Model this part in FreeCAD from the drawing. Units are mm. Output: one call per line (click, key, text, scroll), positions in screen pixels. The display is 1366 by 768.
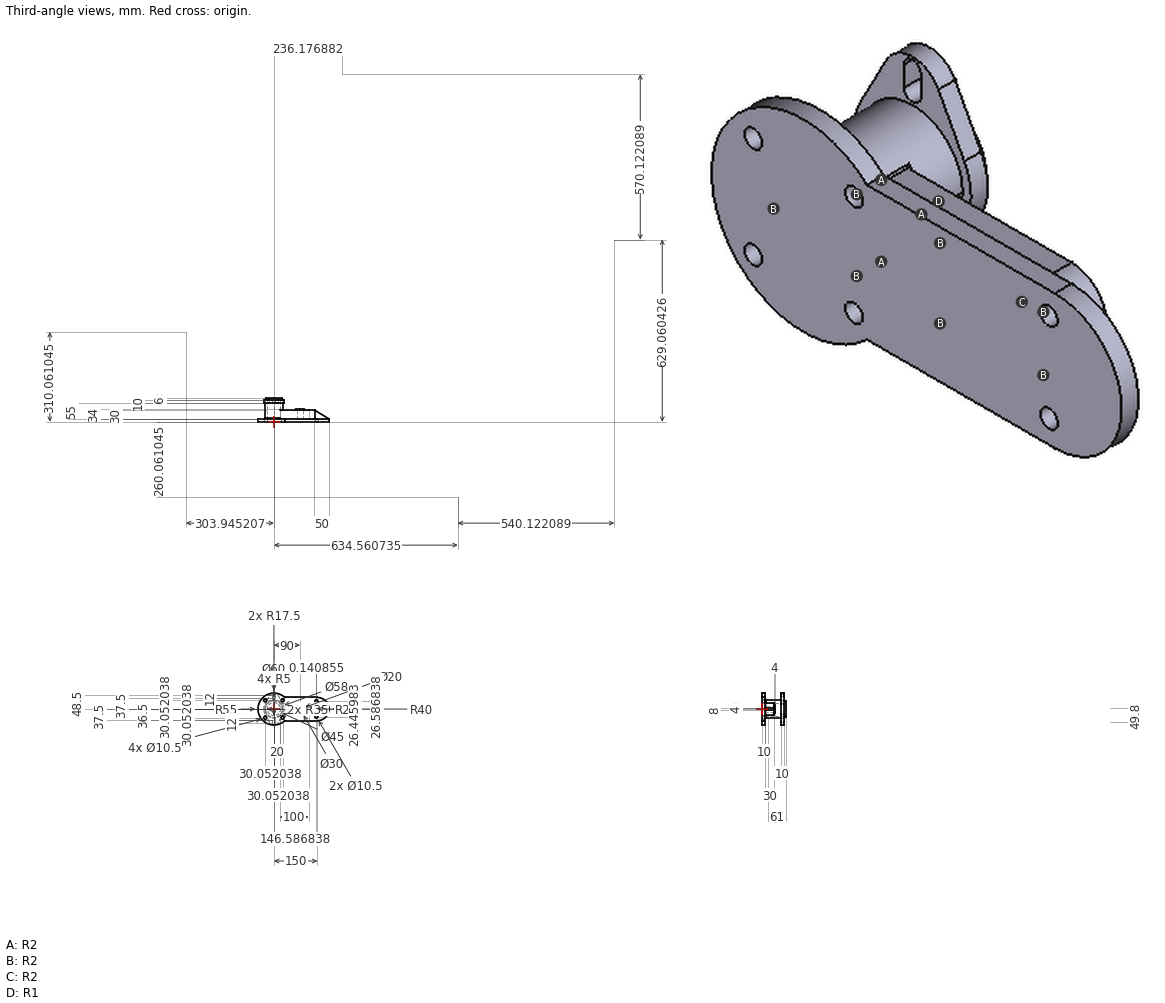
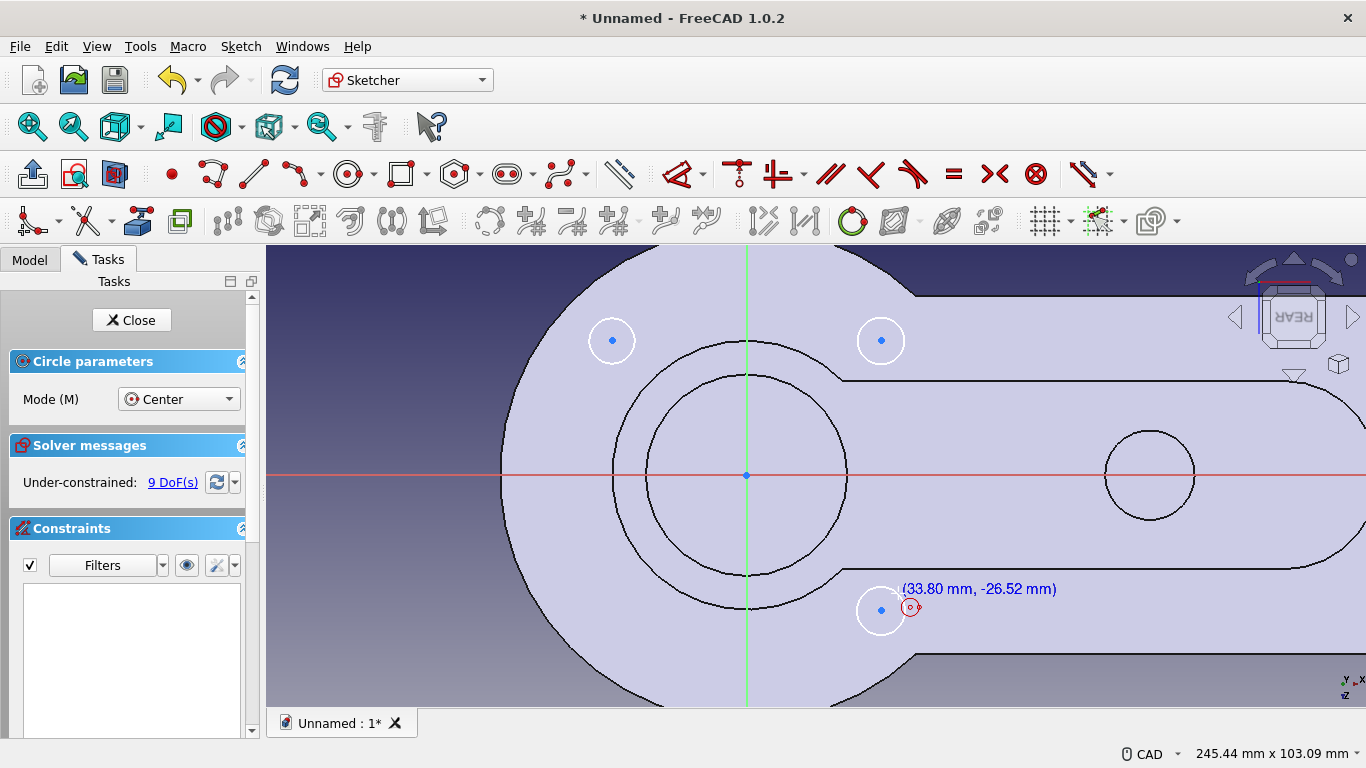
click(612, 610)
click(628, 593)
key(Escape)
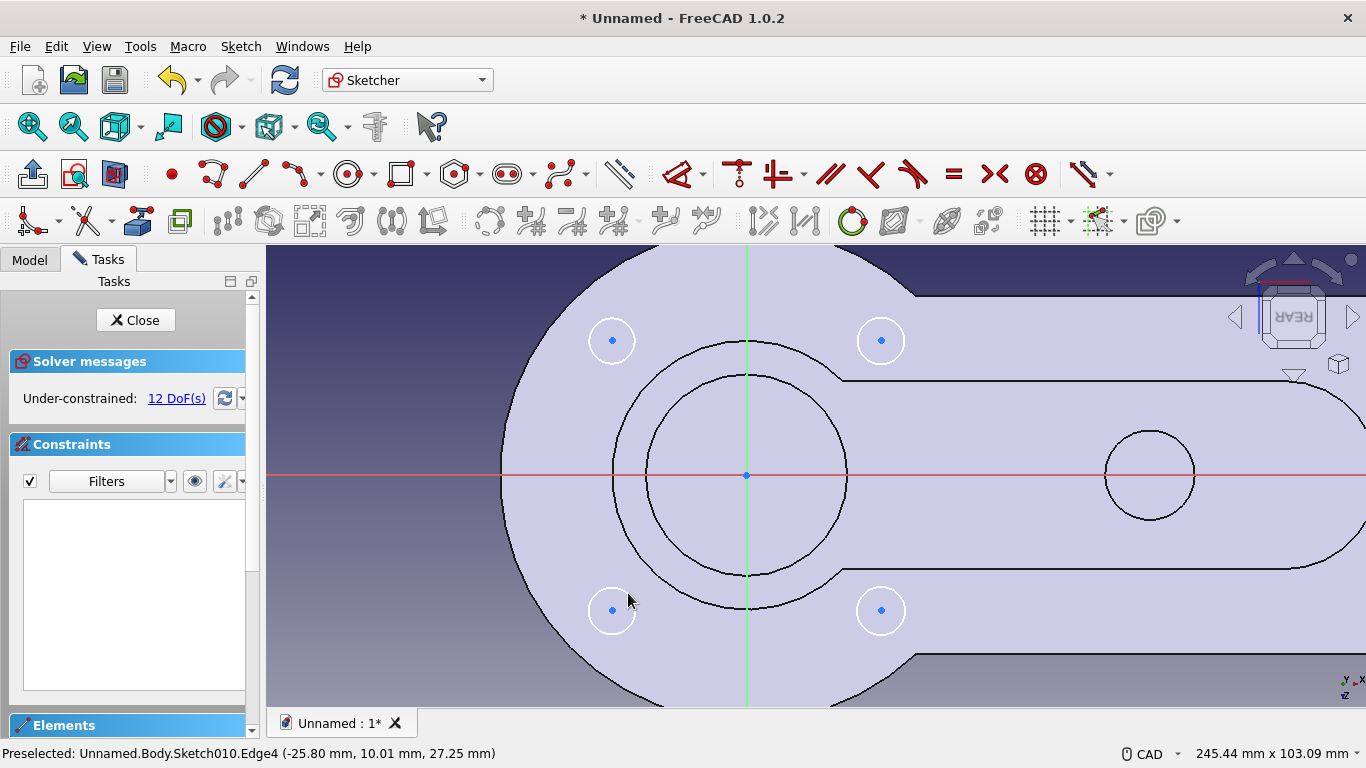
click(628, 325)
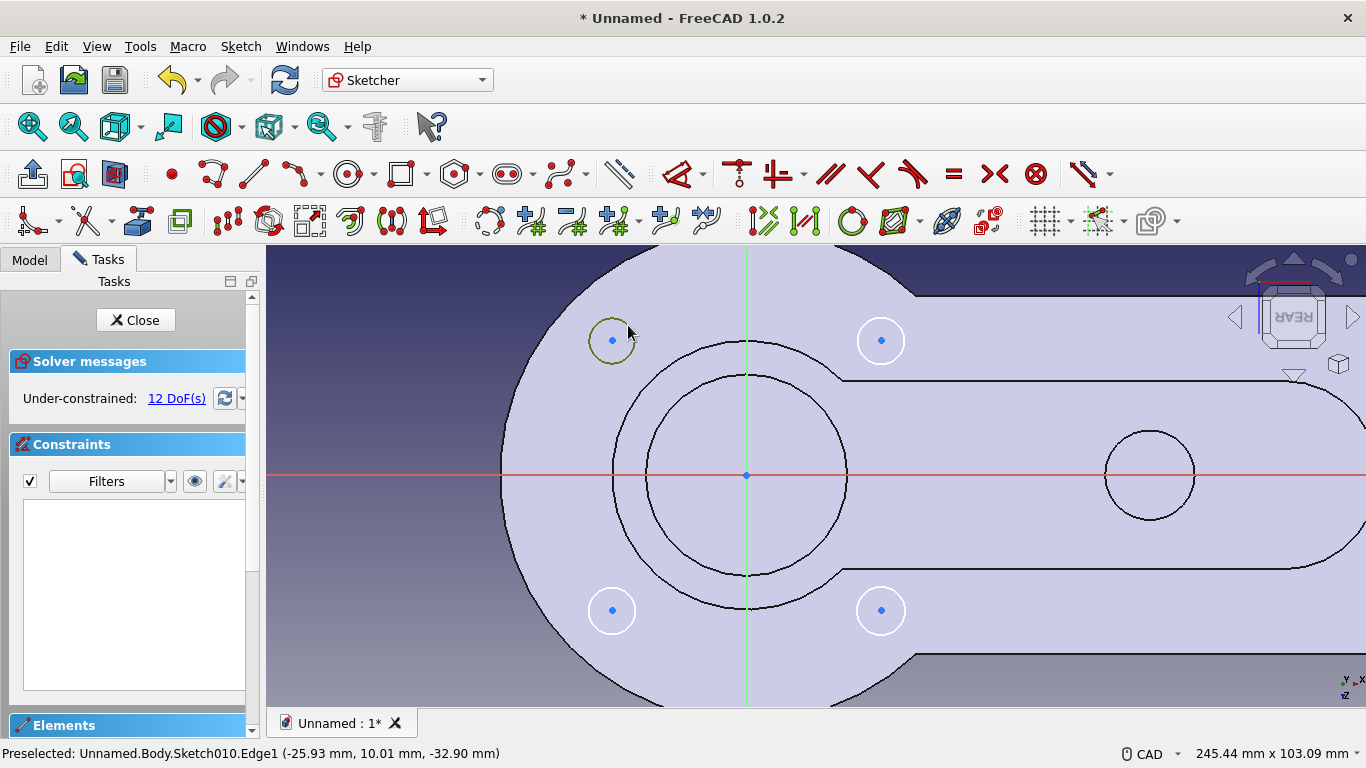
click(897, 324)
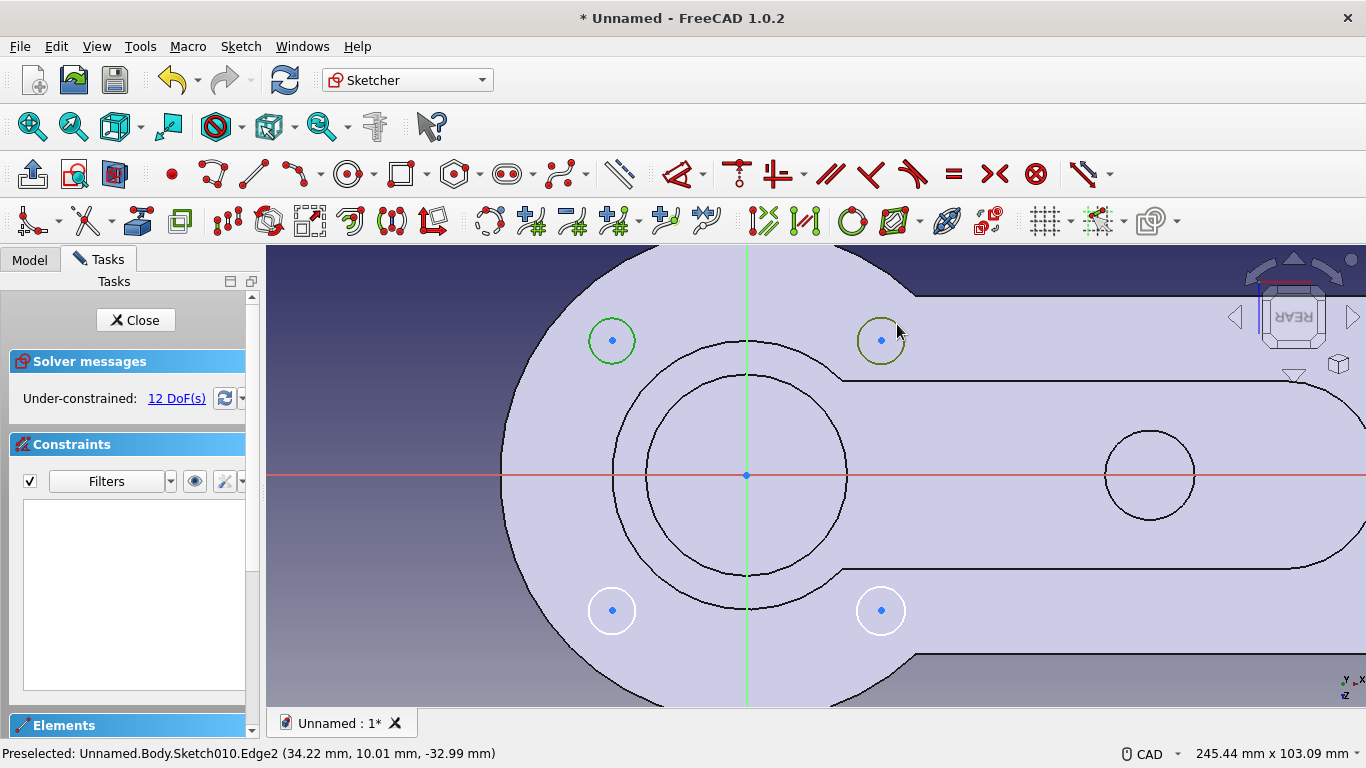
click(898, 594)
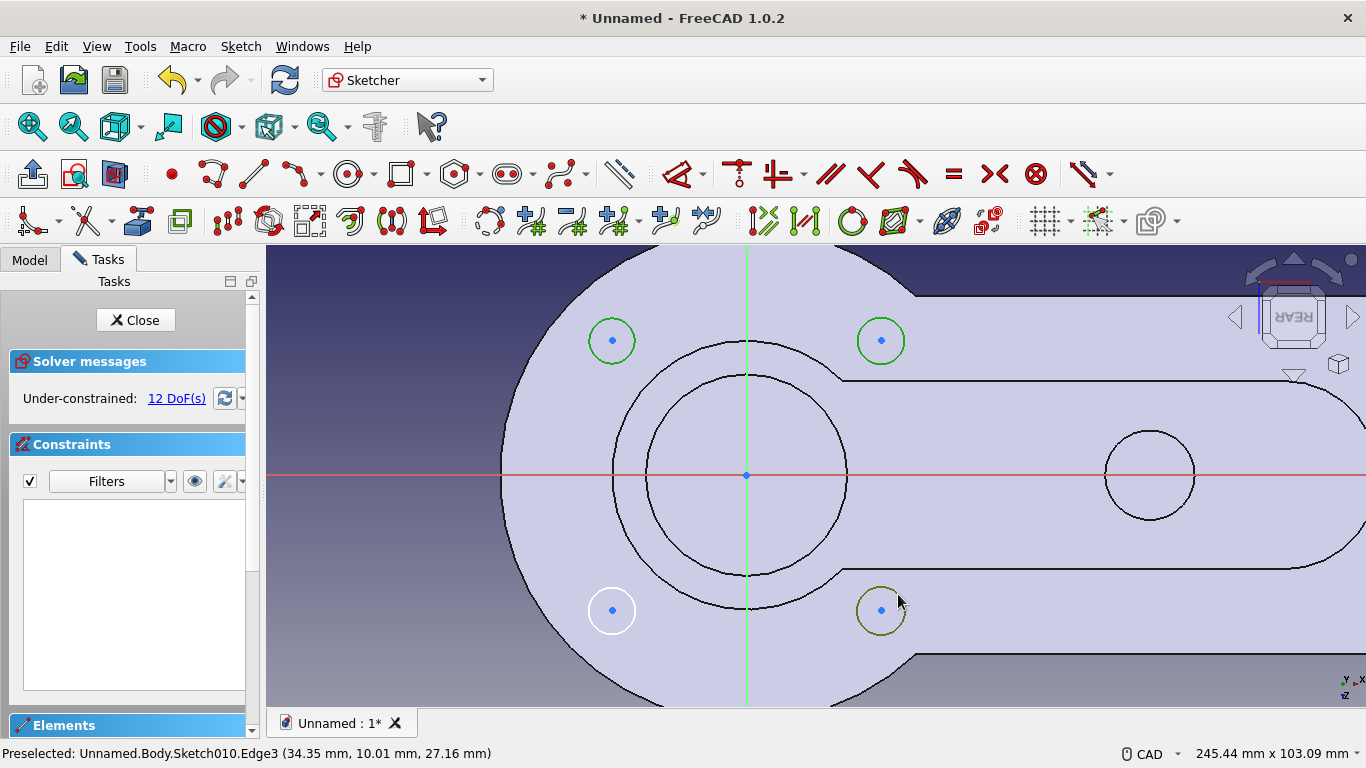
click(628, 594)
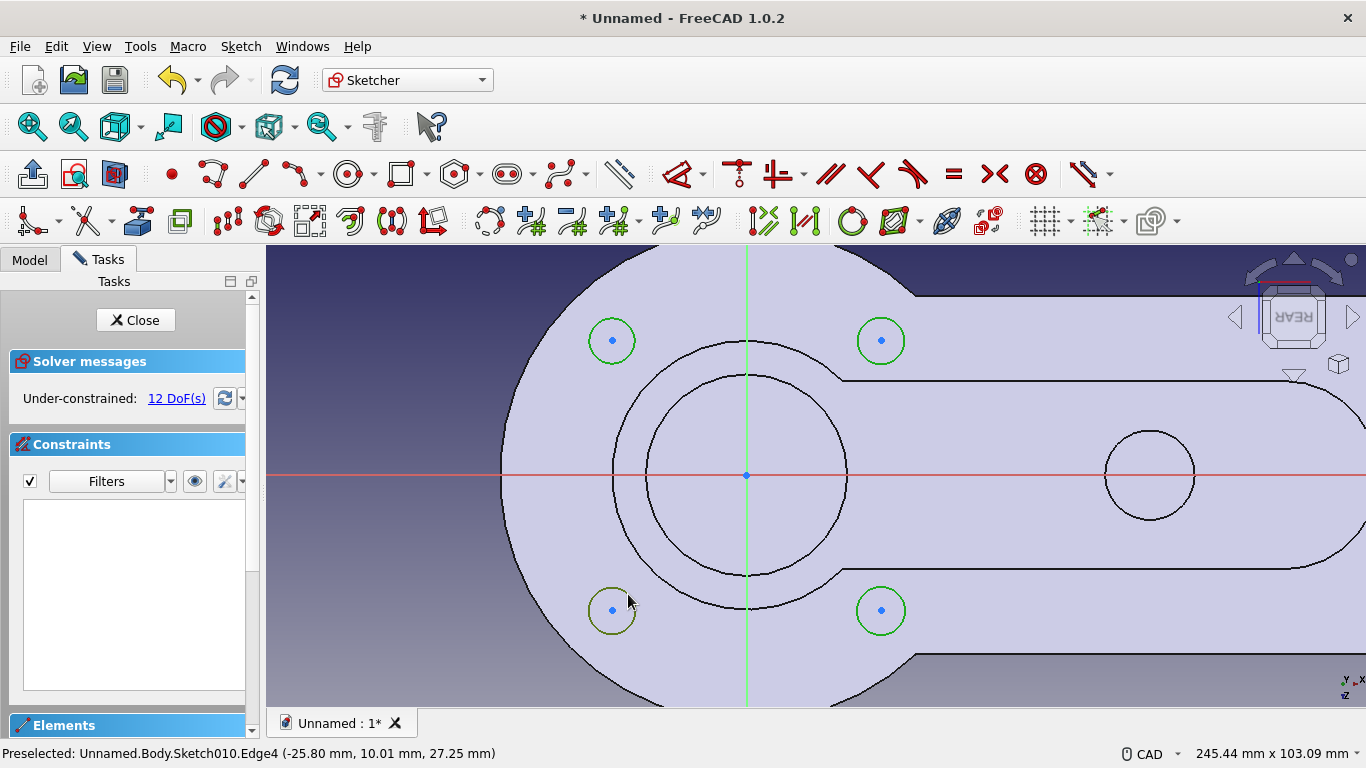
key(e)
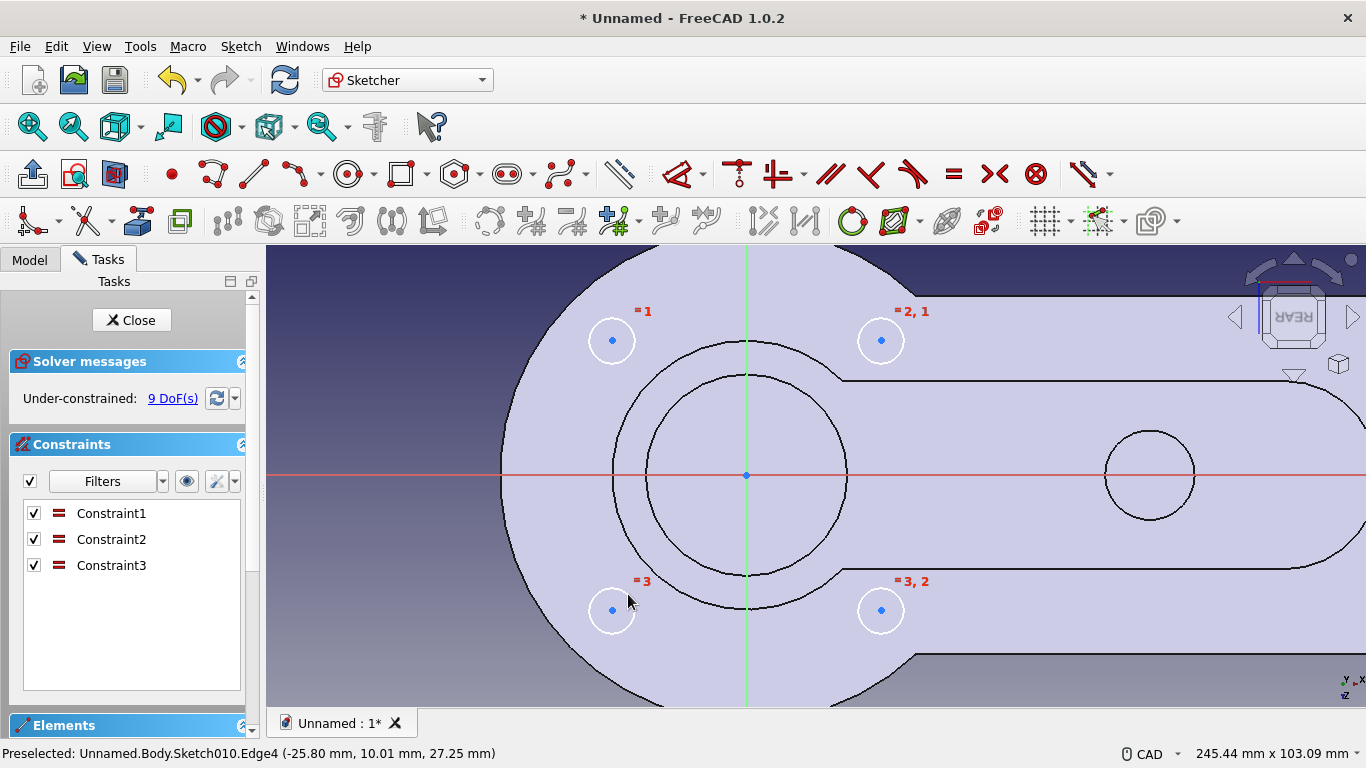
click(612, 341)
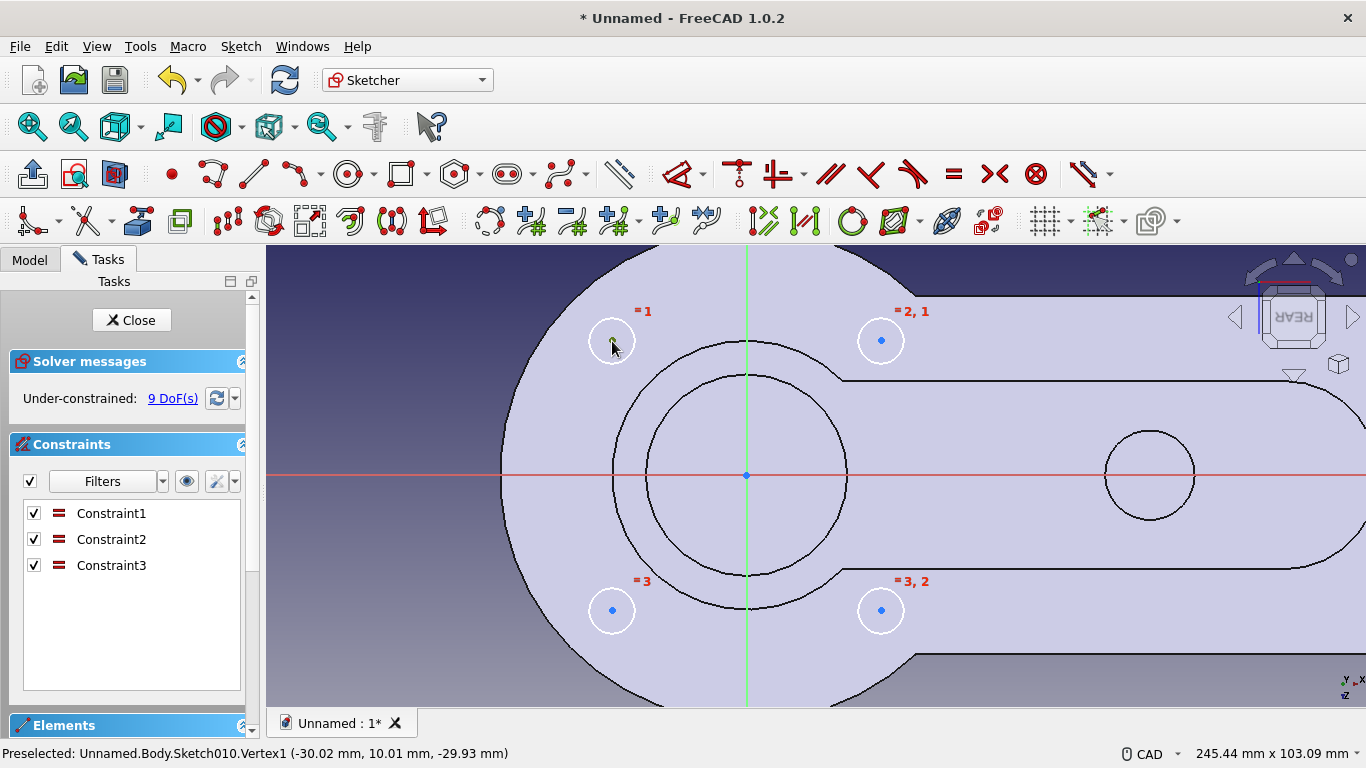
click(881, 341)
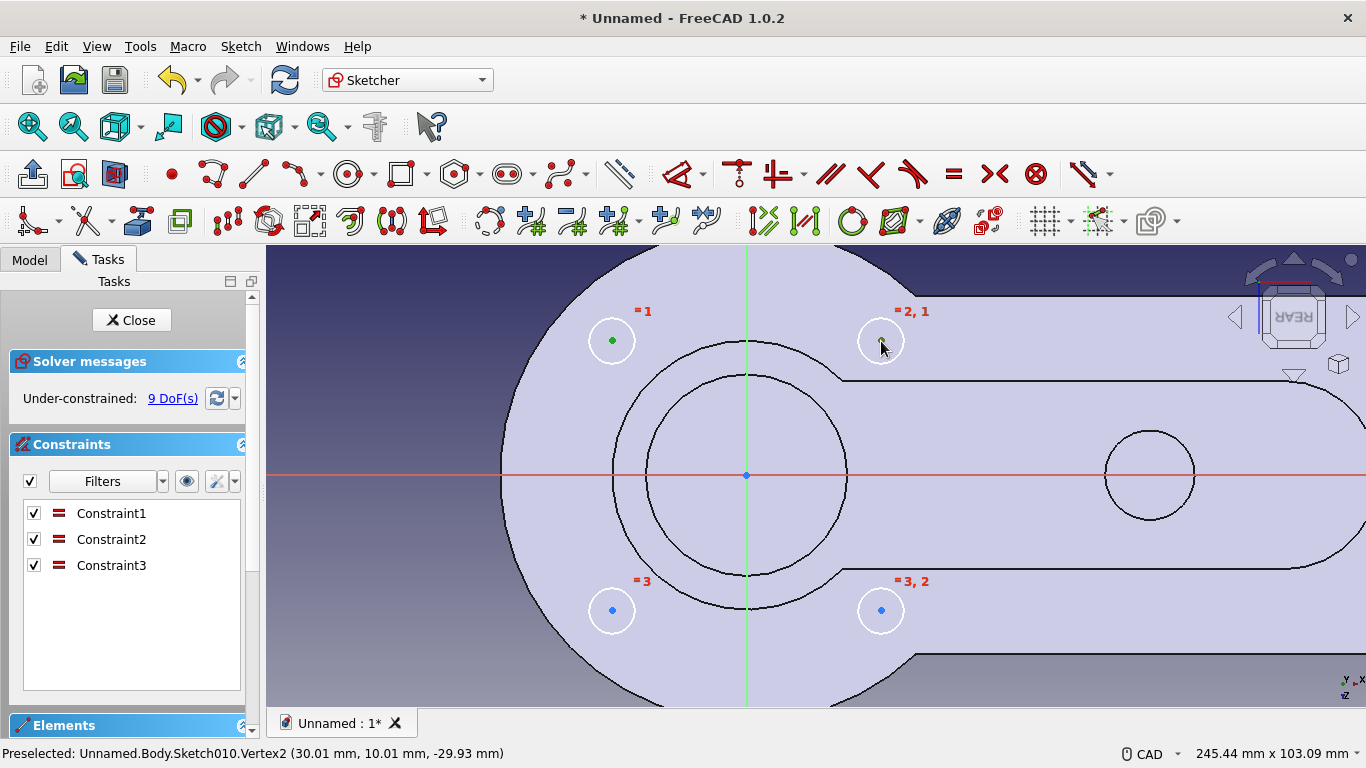
click(804, 174)